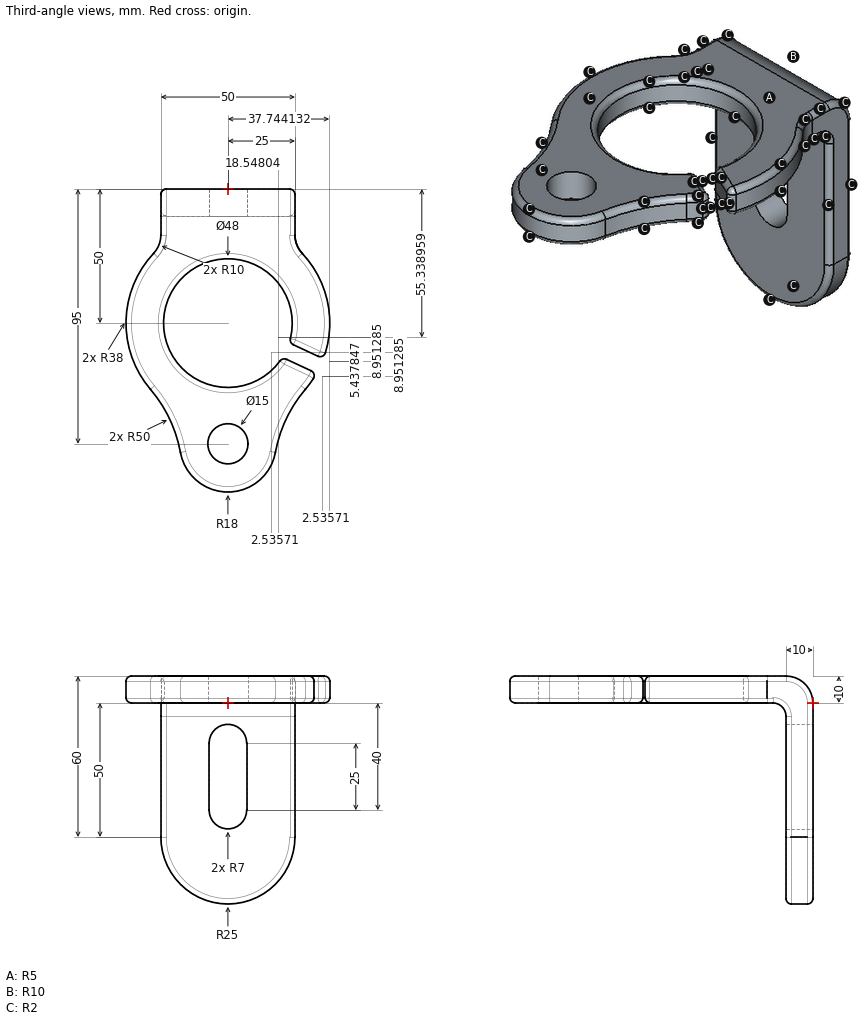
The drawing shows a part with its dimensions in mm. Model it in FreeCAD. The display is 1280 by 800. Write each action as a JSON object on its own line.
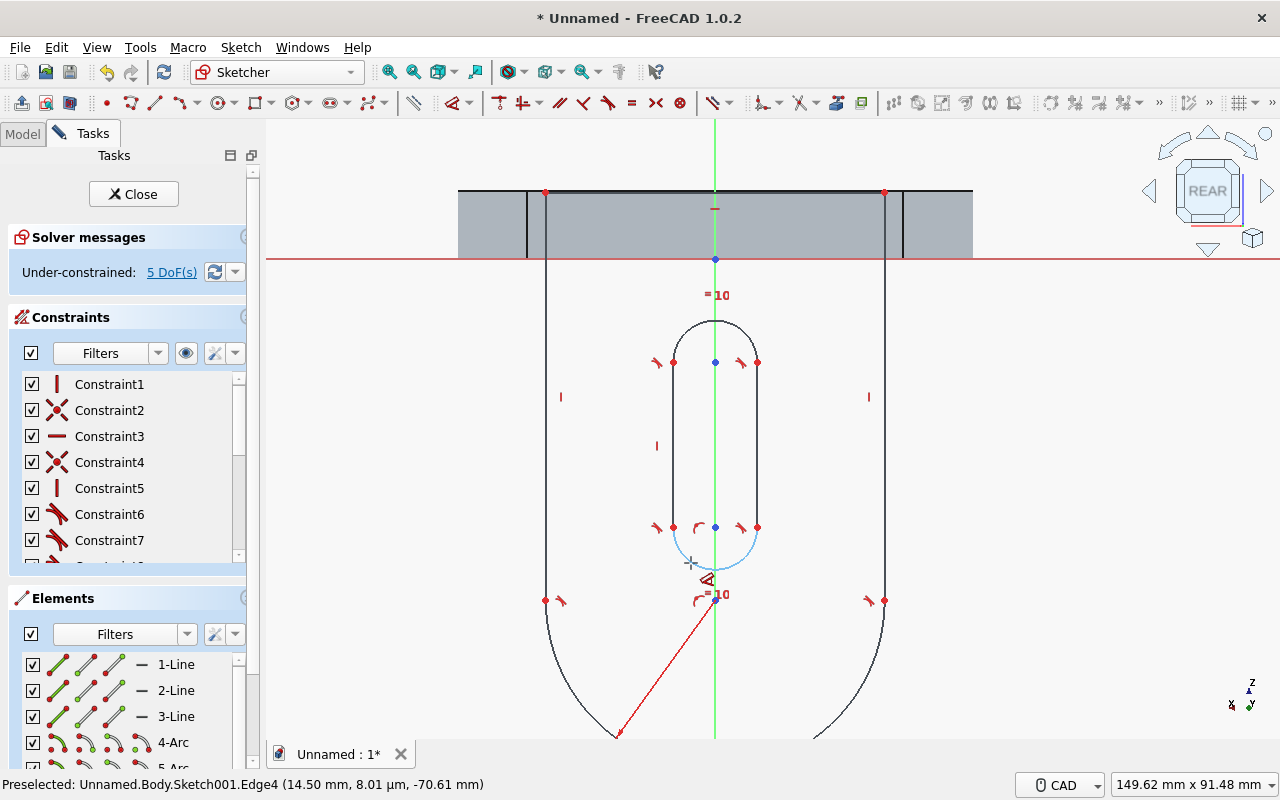
{"action": "left_click", "coordinate": [691, 562]}
{"action": "left_click", "coordinate": [672, 588]}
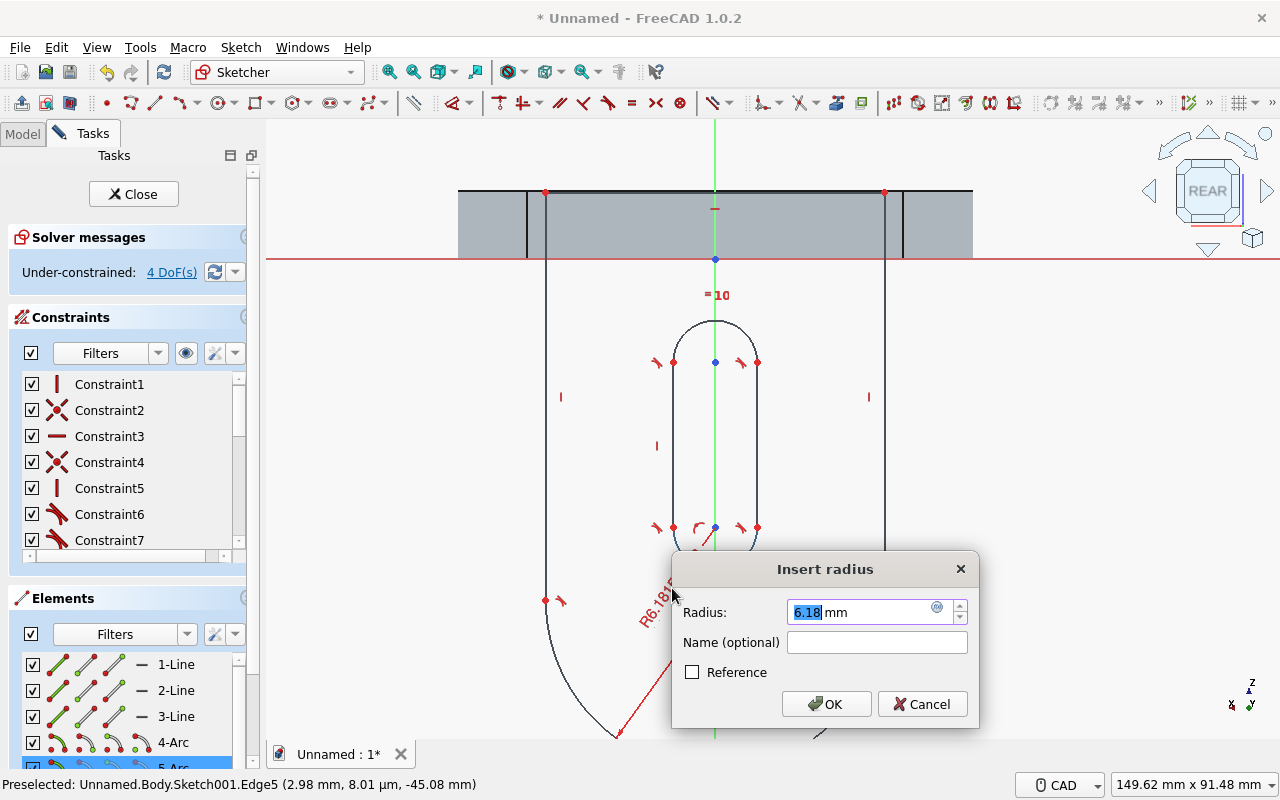
{"action": "type", "text": "7"}
{"action": "key", "text": "Return"}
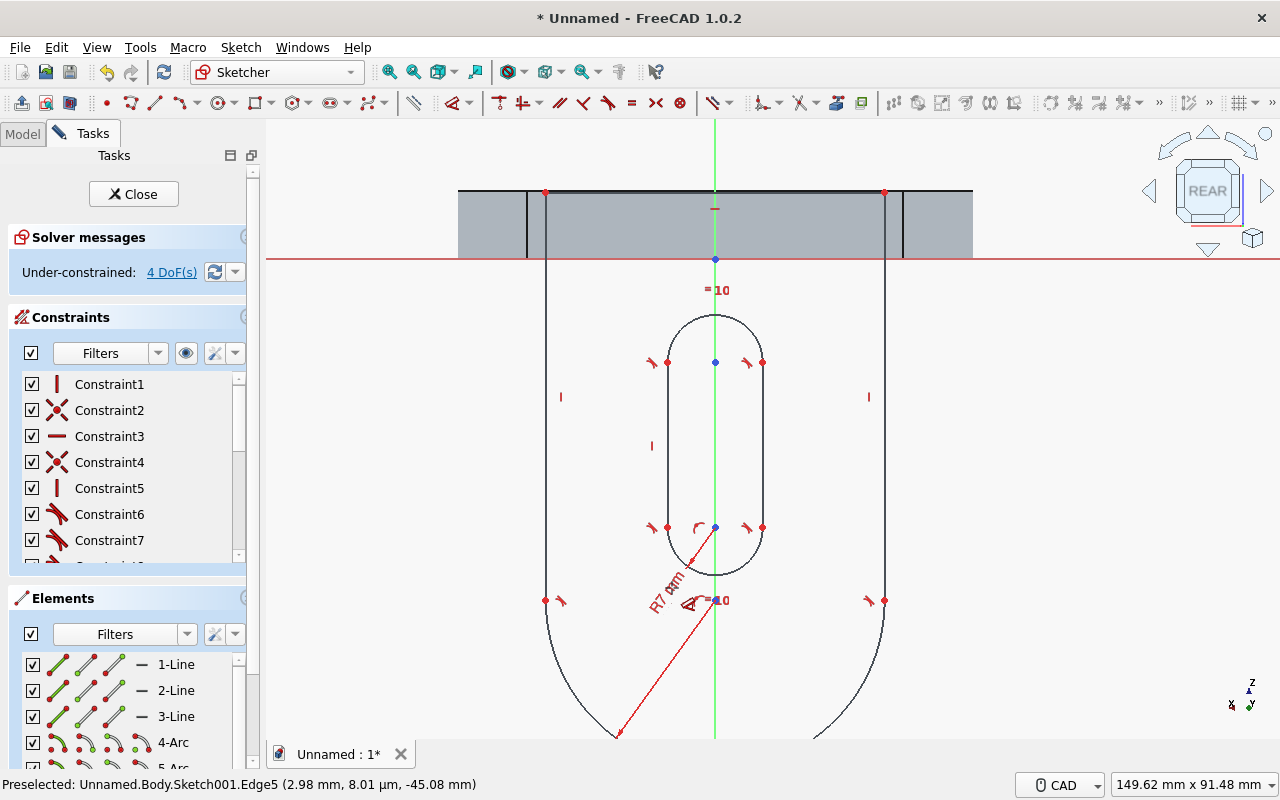
{"action": "left_click", "coordinate": [885, 478]}
{"action": "left_click", "coordinate": [919, 397]}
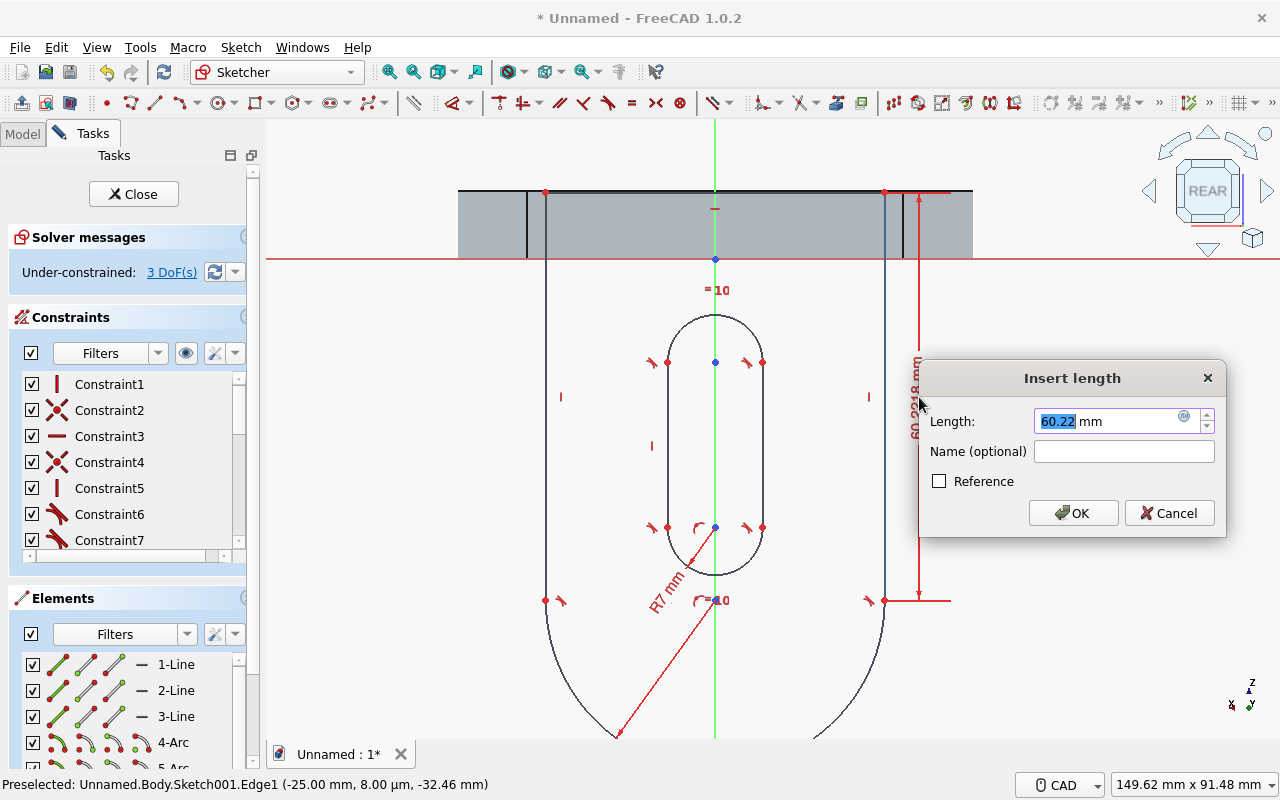
{"action": "type", "text": "60"}
{"action": "key", "text": "Return"}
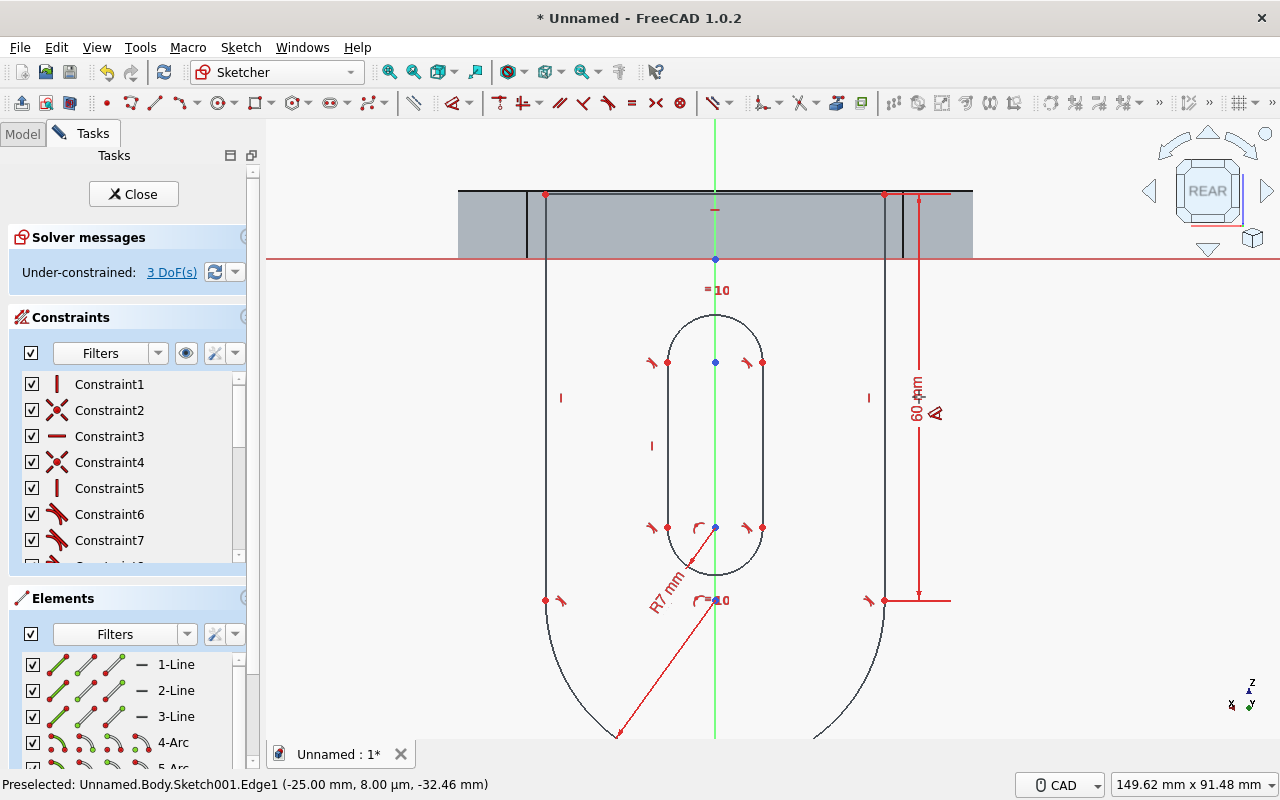
{"action": "left_click", "coordinate": [668, 478]}
{"action": "left_click", "coordinate": [634, 445]}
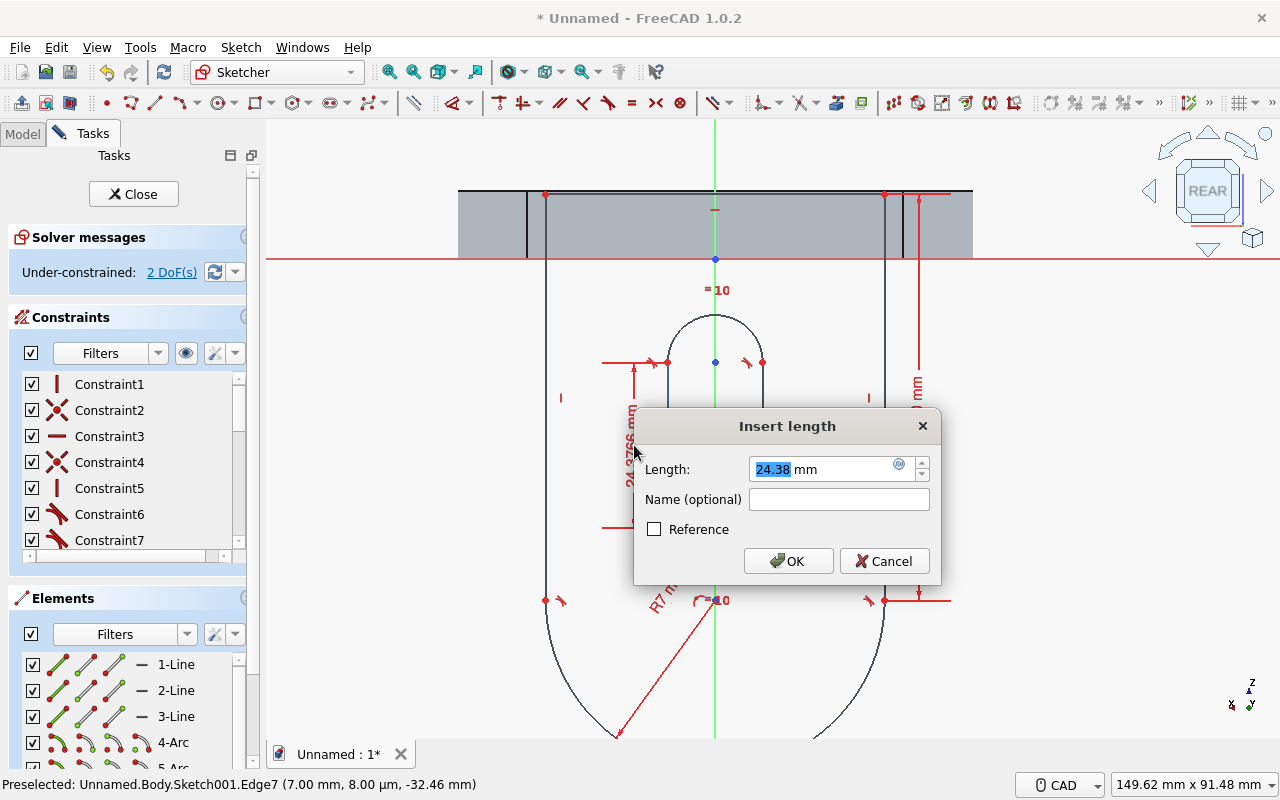
{"action": "type", "text": "25"}
{"action": "key", "text": "Return"}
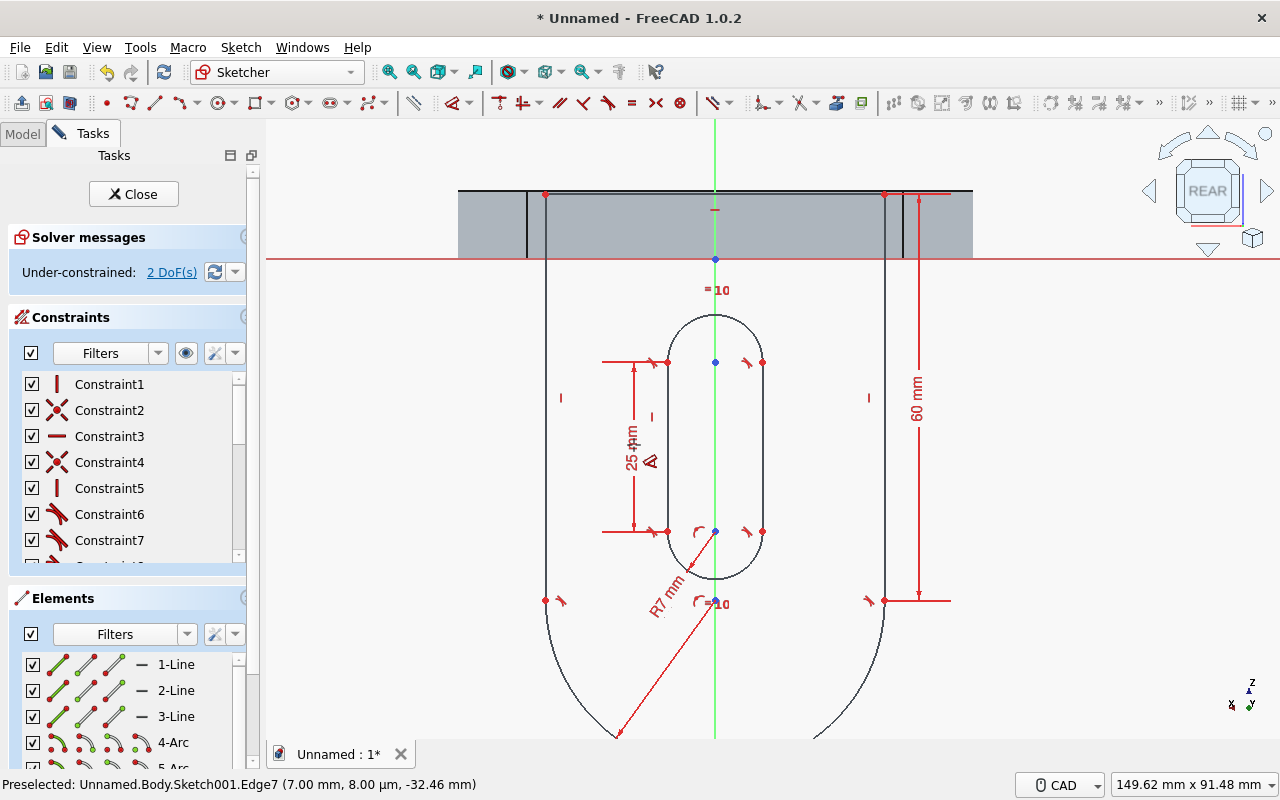
{"action": "left_click", "coordinate": [885, 601]}
{"action": "left_click", "coordinate": [919, 430]}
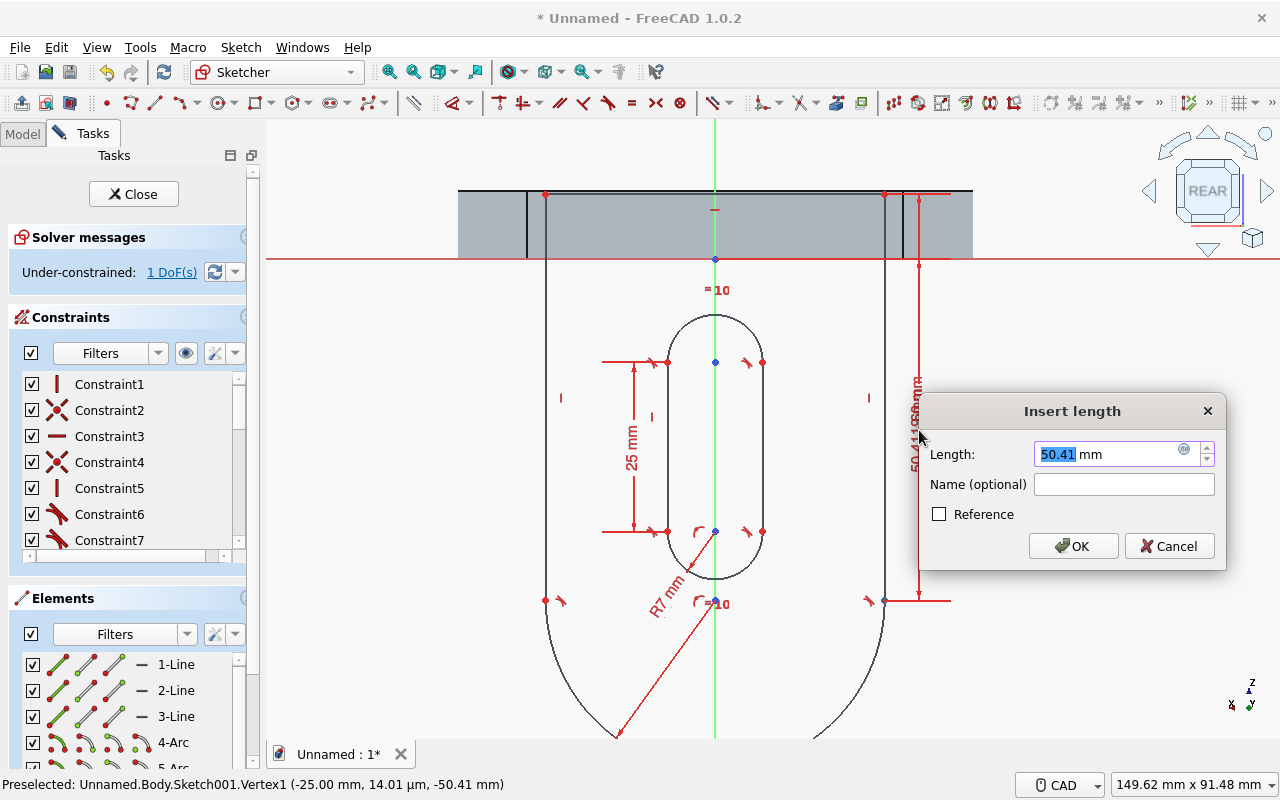
{"action": "type", "text": "50"}
{"action": "key", "text": "Return"}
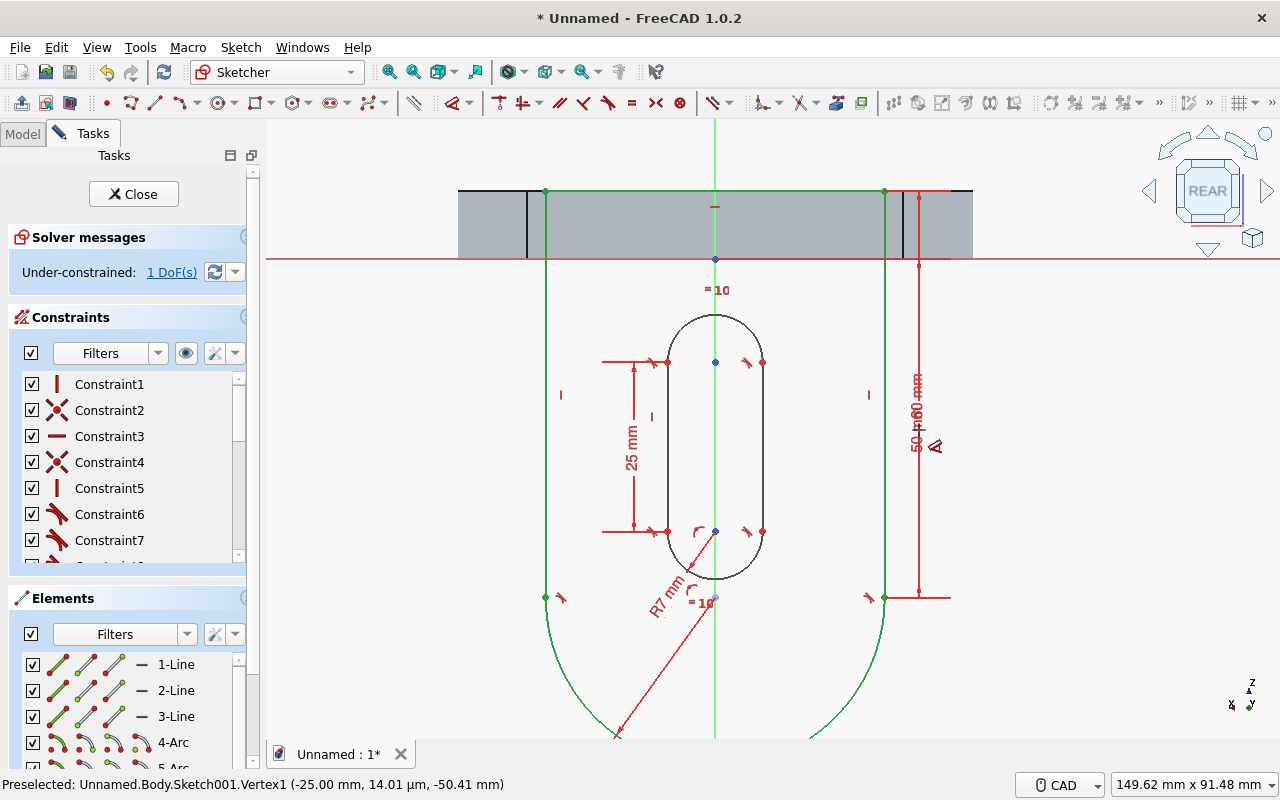
{"action": "left_click", "coordinate": [668, 532]}
{"action": "left_click", "coordinate": [634, 395]}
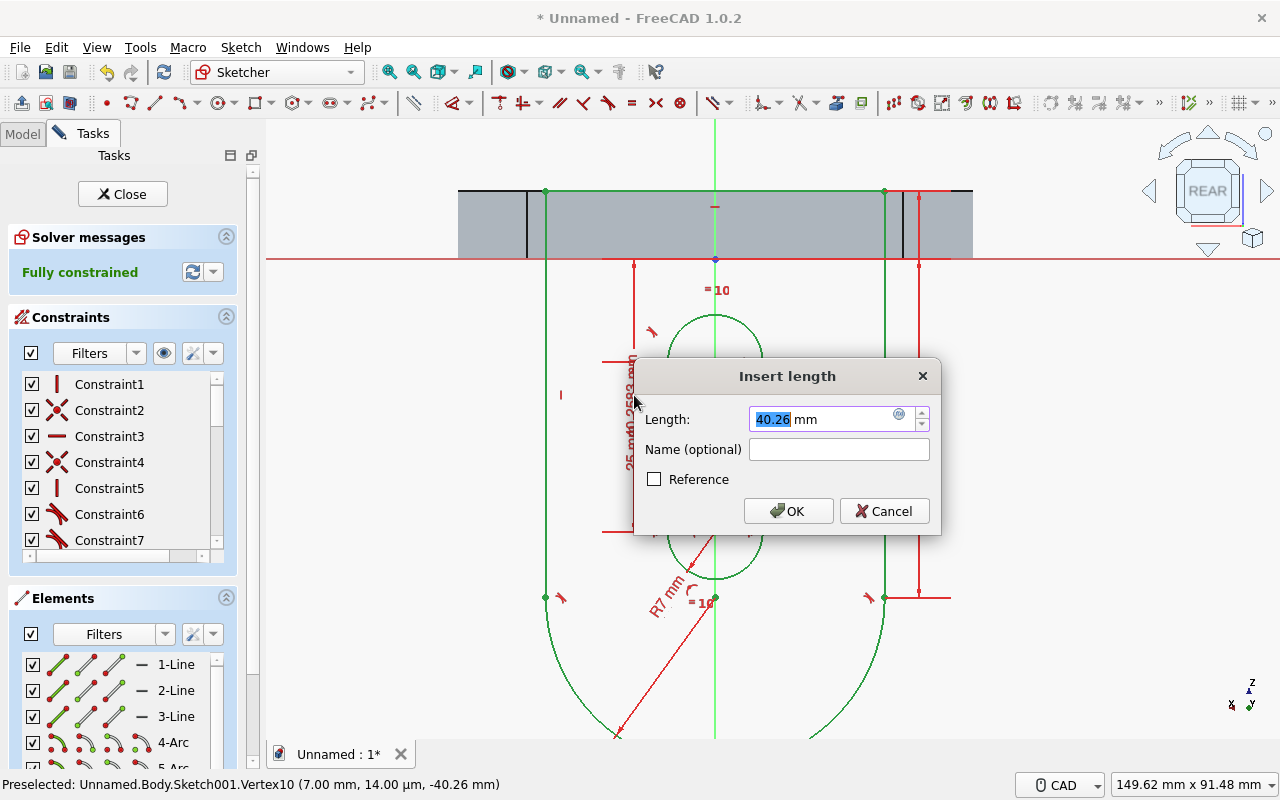
{"action": "type", "text": "40"}
{"action": "key", "text": "Return"}
{"action": "key", "text": "Escape"}